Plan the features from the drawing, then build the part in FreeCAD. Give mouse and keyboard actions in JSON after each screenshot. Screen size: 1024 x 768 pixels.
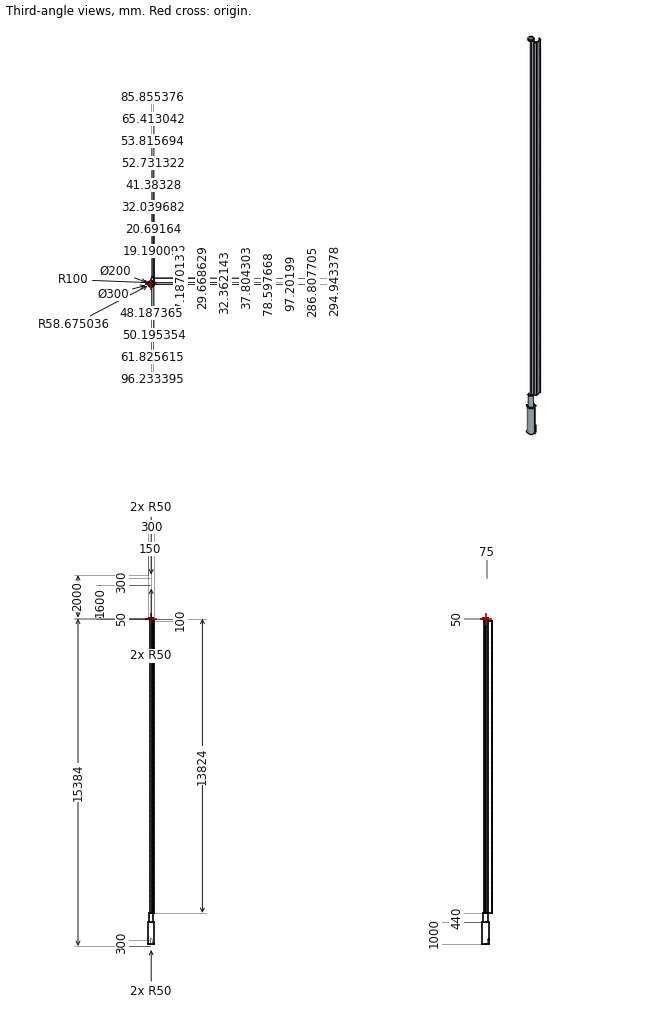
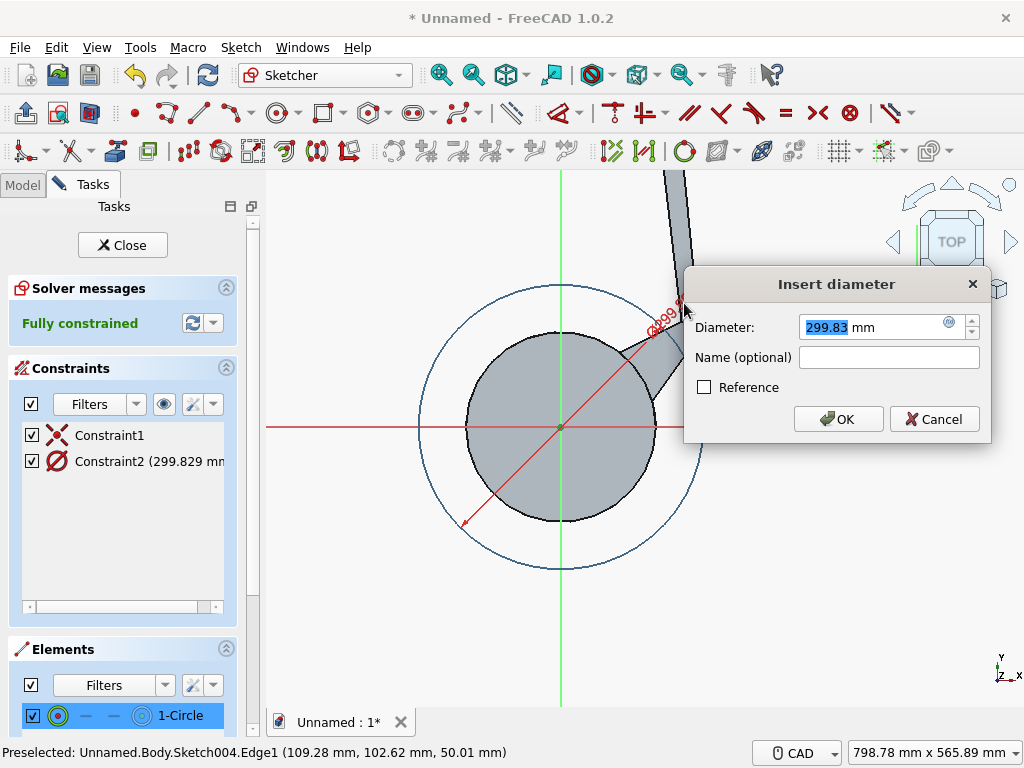
{"action": "type", "text": "300"}
{"action": "key", "text": "Return"}
{"action": "key", "text": "Escape"}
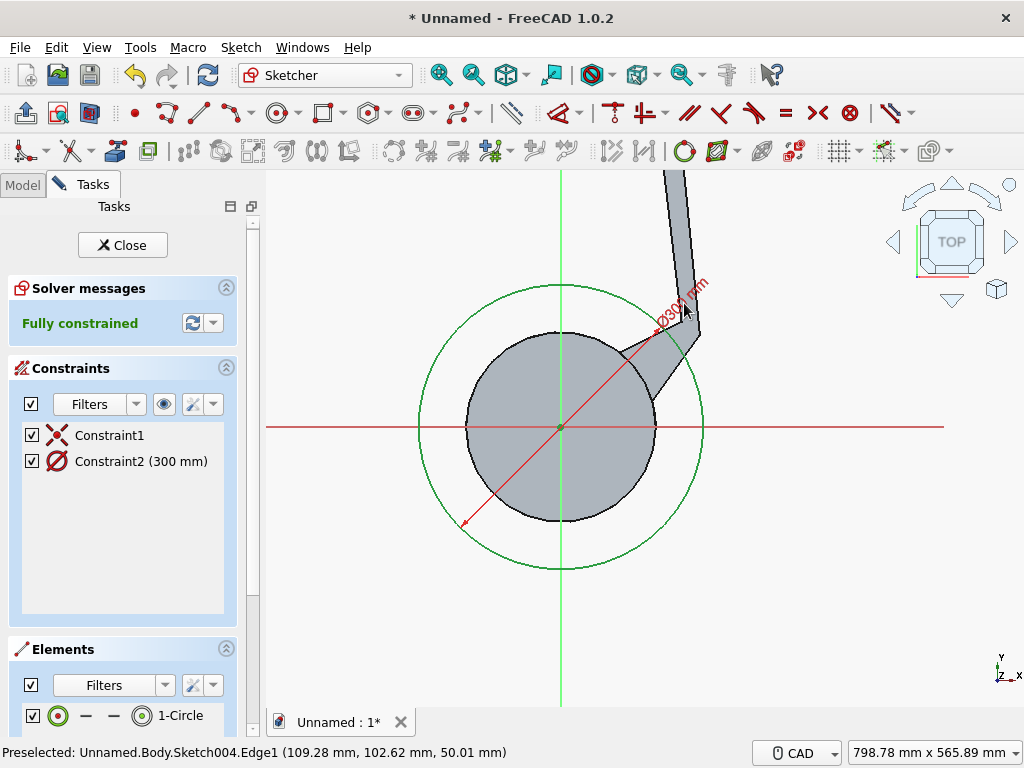
{"action": "left_click", "coordinate": [123, 245]}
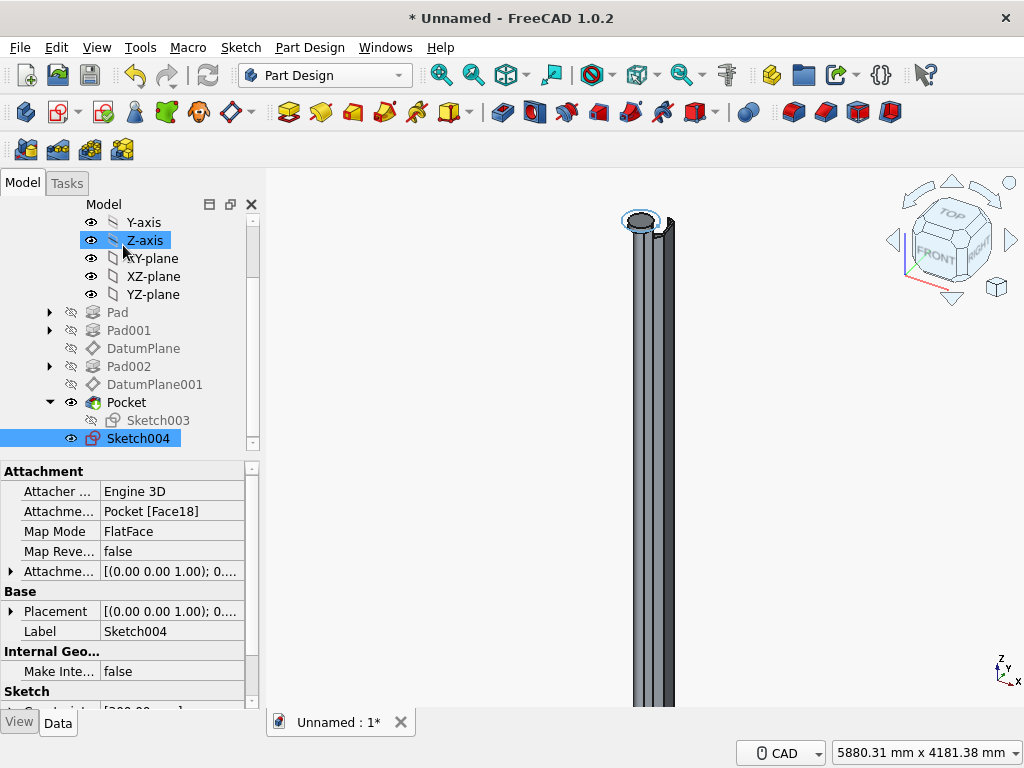
{"action": "left_click", "coordinate": [290, 112]}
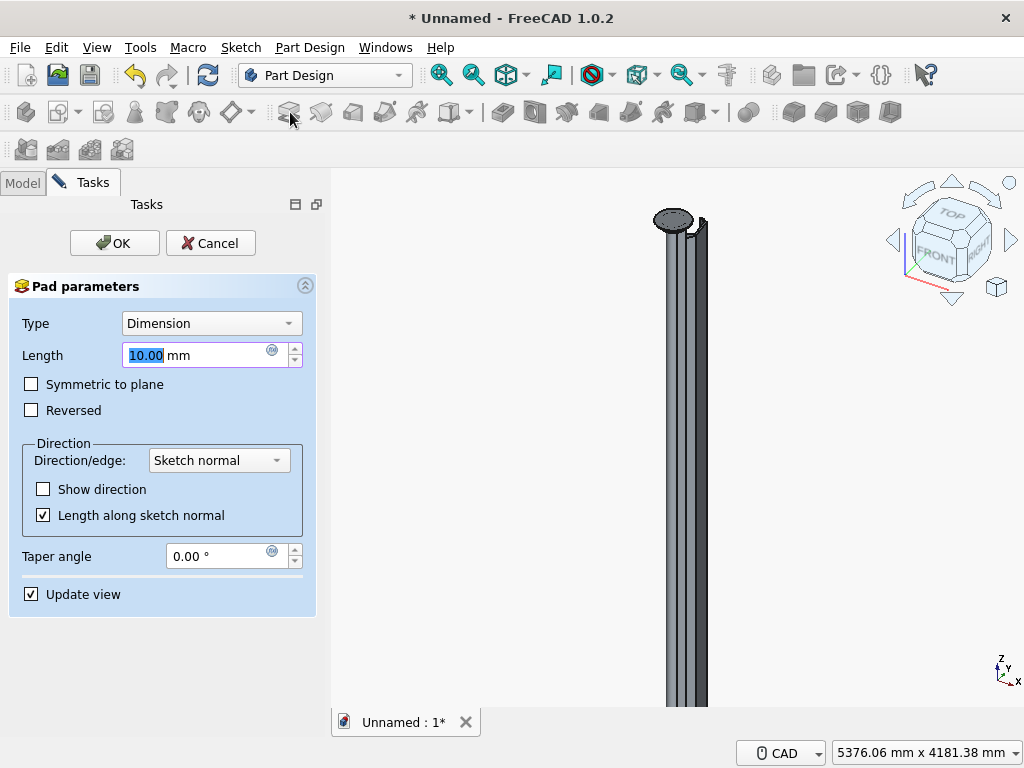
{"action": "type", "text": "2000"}
{"action": "key", "text": "Tab"}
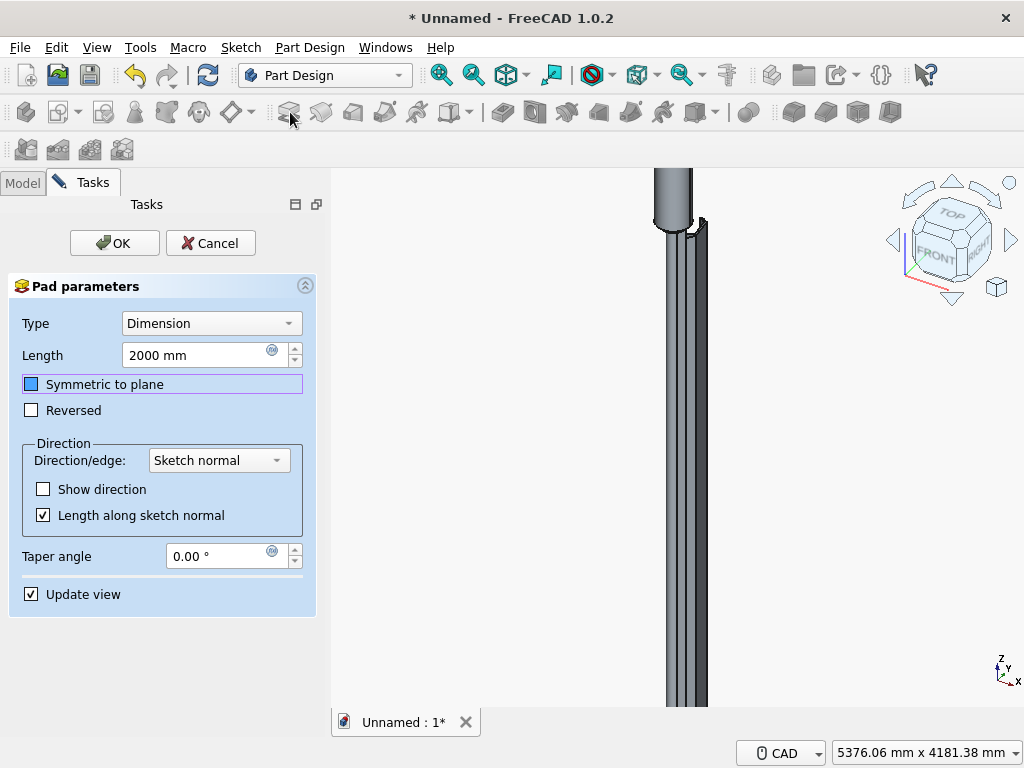
{"action": "left_click", "coordinate": [115, 243]}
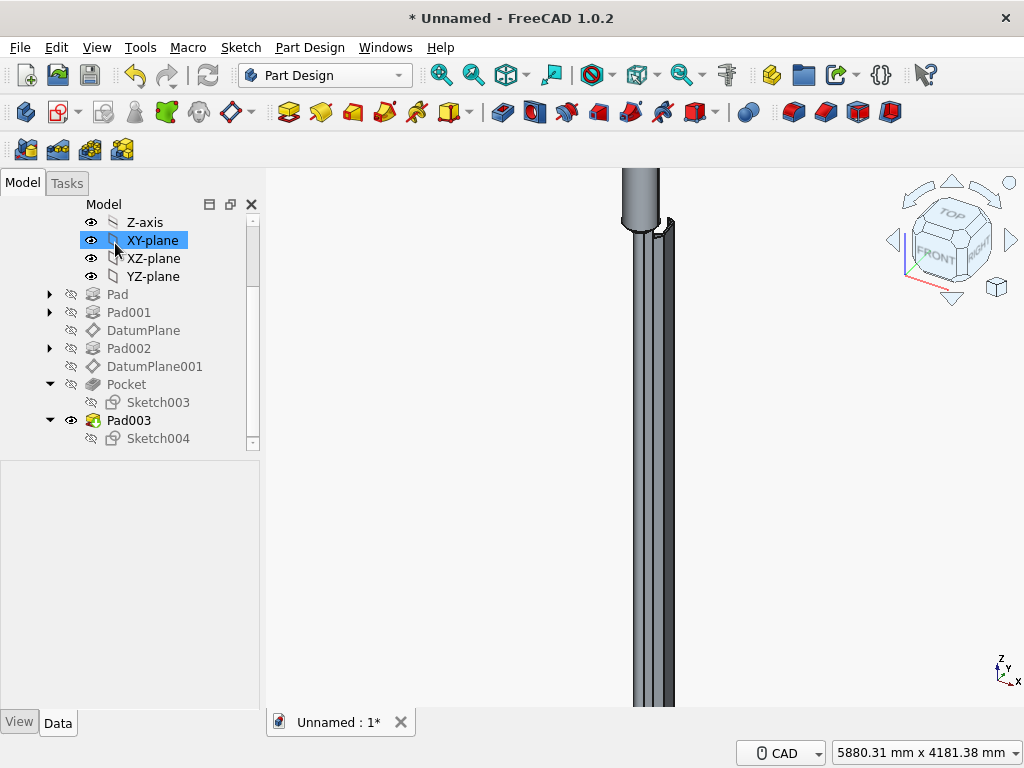
{"action": "left_click", "coordinate": [442, 76]}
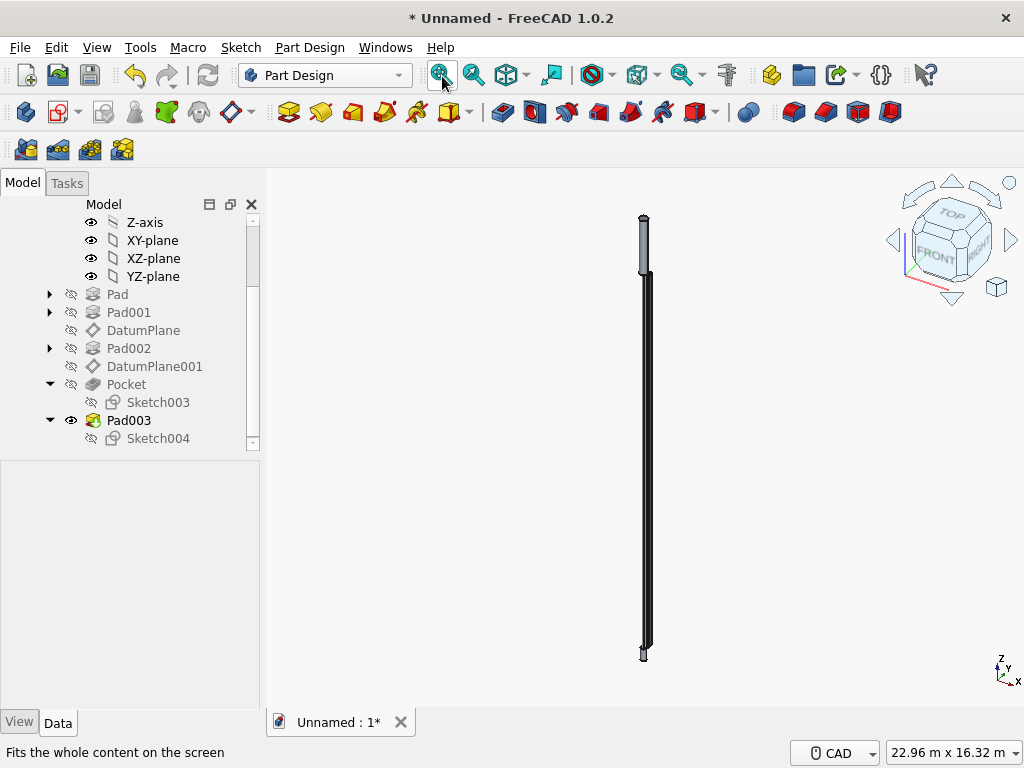
{"action": "left_click", "coordinate": [58, 112]}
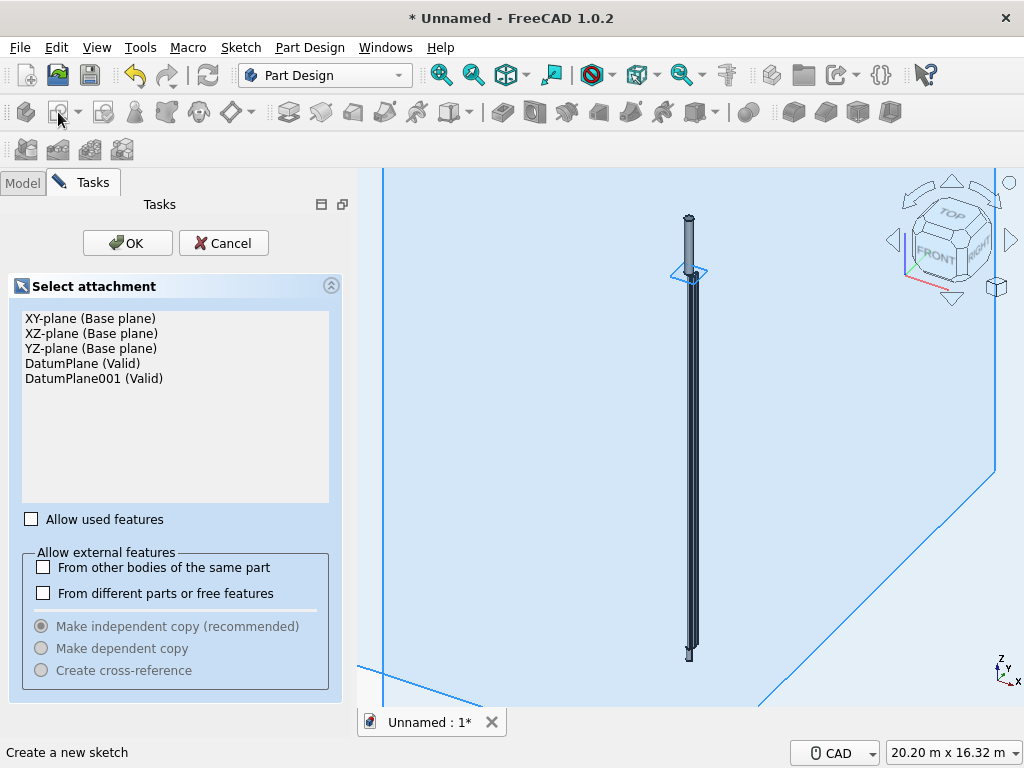
{"action": "left_click", "coordinate": [82, 334]}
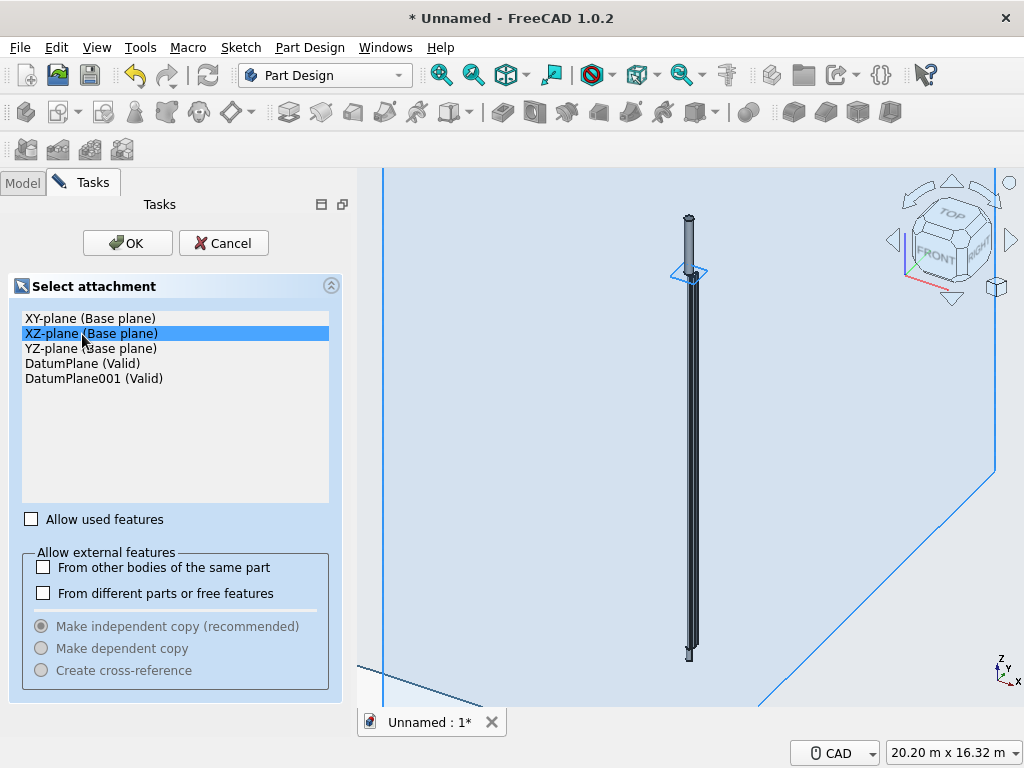
{"action": "left_click", "coordinate": [128, 243]}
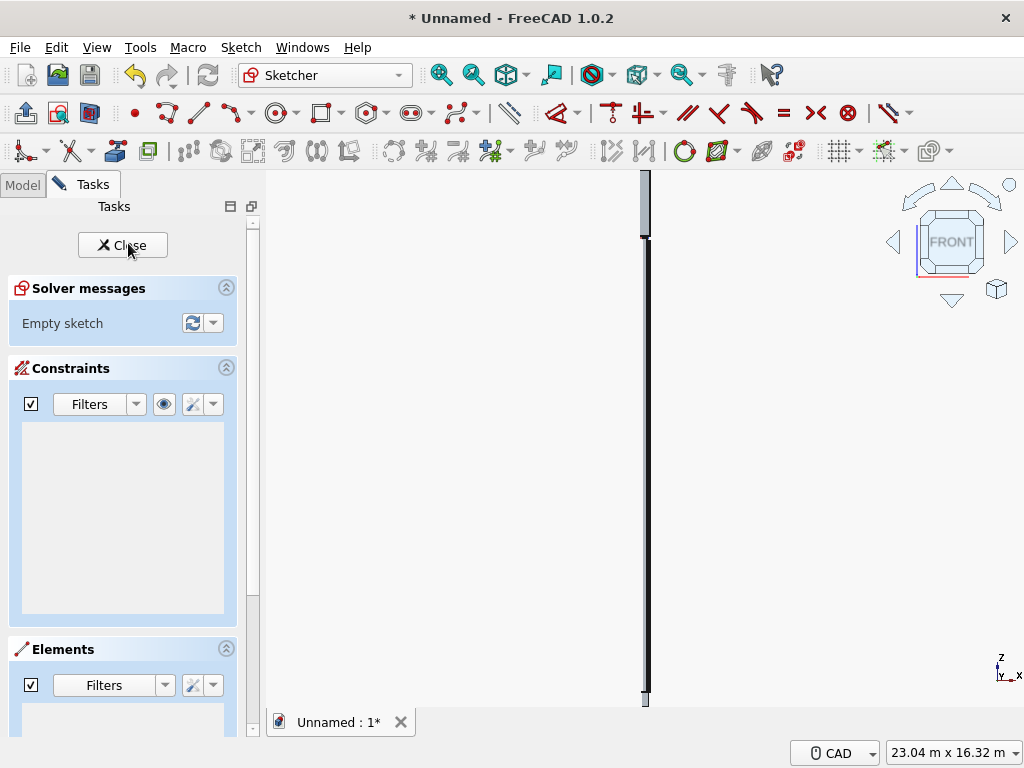
{"action": "left_click", "coordinate": [90, 114]}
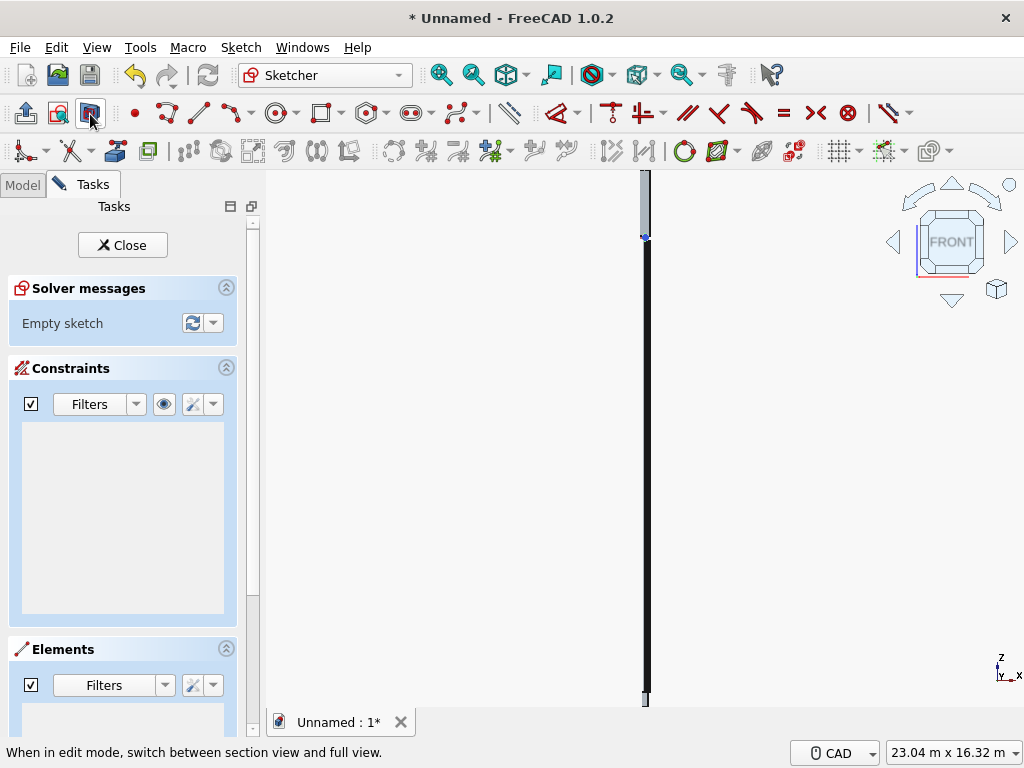
{"action": "scroll", "coordinate": [576, 438], "scroll_direction": "down", "scroll_amount": 5}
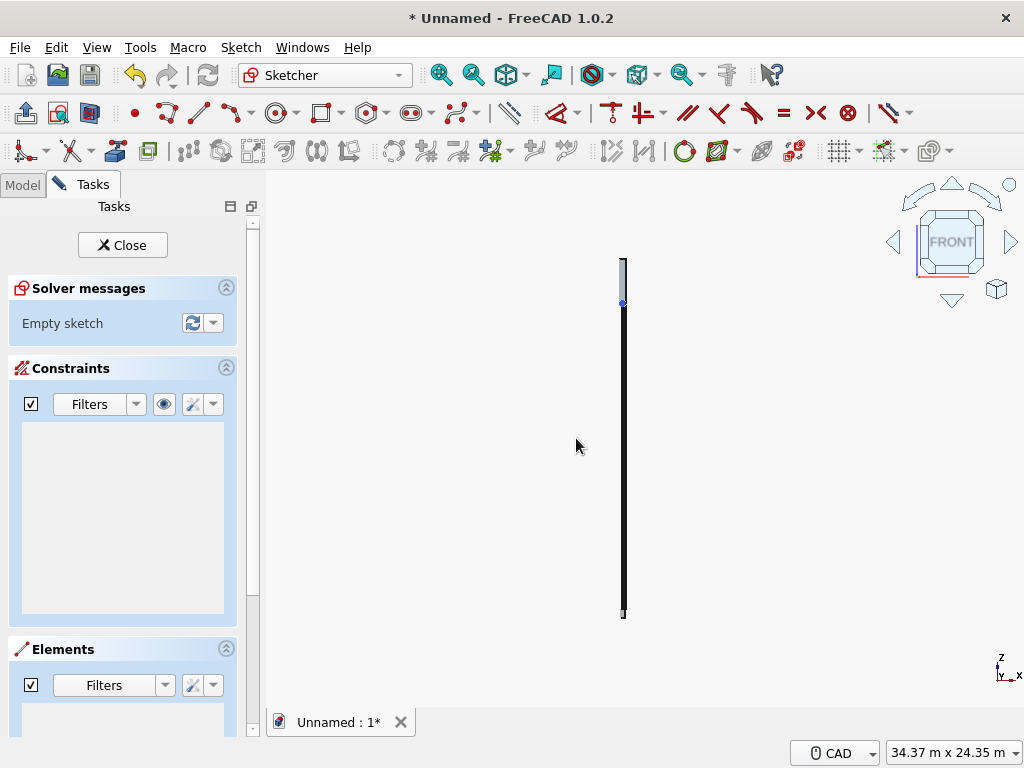
{"action": "scroll", "coordinate": [603, 338], "scroll_direction": "up", "scroll_amount": 15}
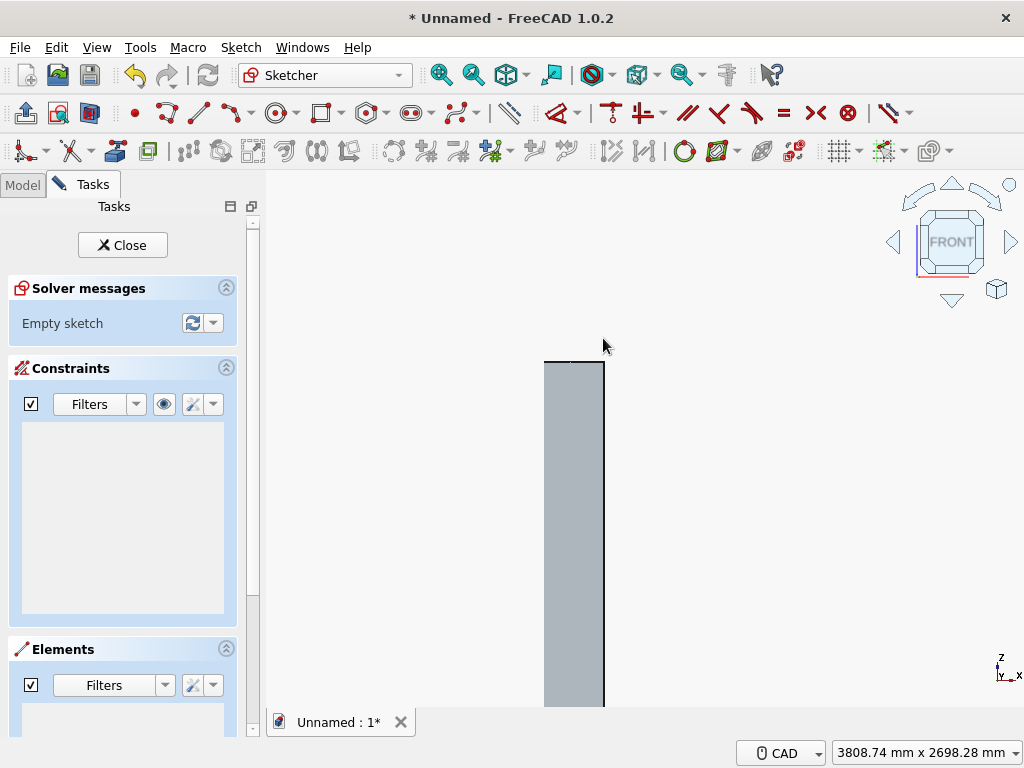
{"action": "scroll", "coordinate": [563, 442], "scroll_direction": "up", "scroll_amount": 6}